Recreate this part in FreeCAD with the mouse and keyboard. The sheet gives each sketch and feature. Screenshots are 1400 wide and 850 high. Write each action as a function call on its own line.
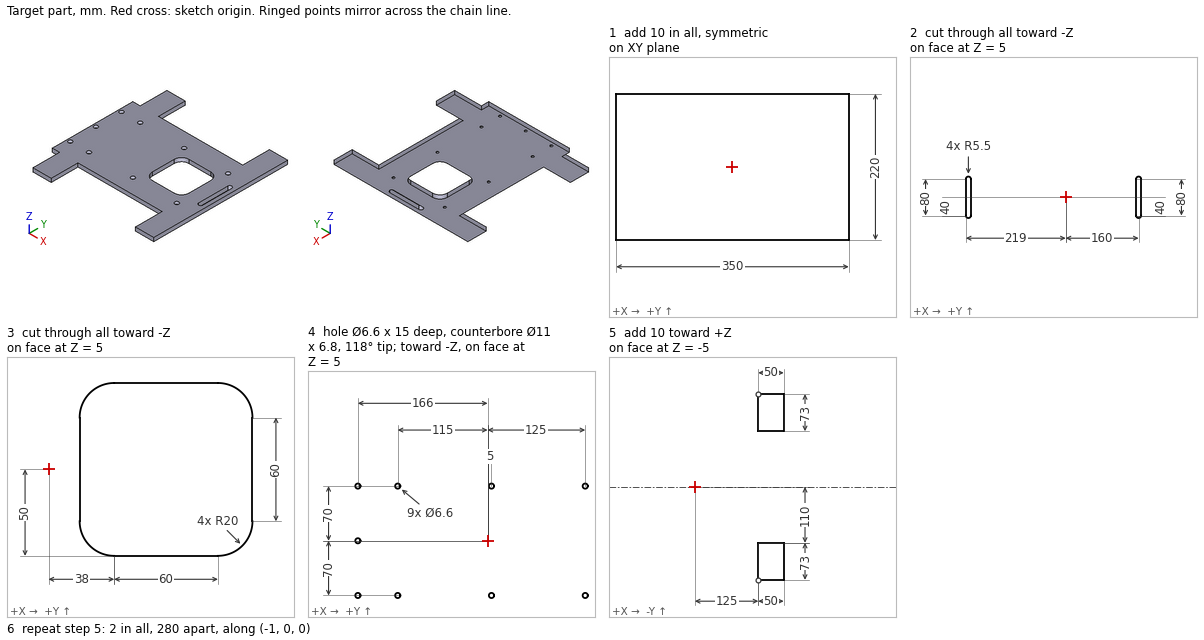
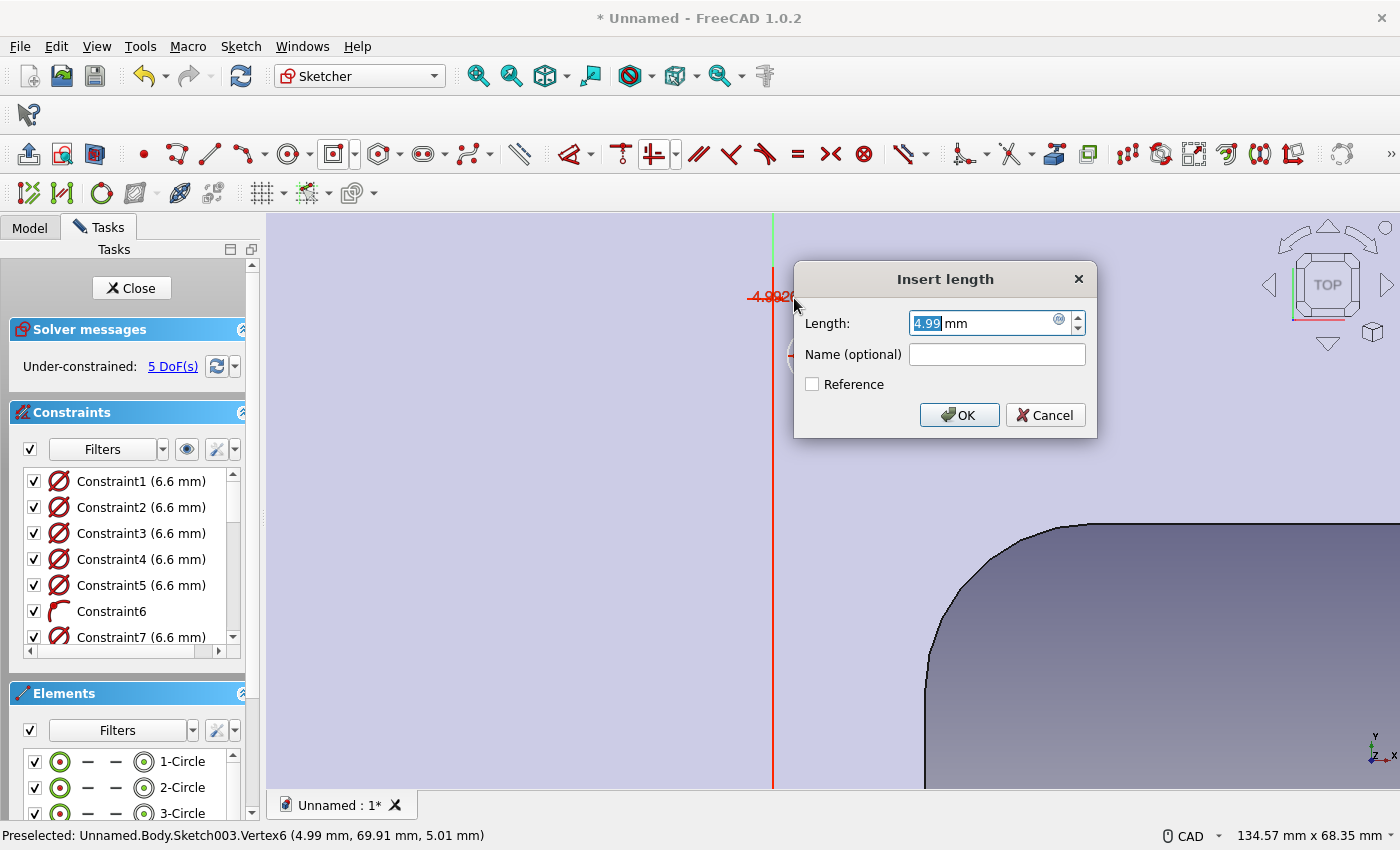
text(5)
key(Return)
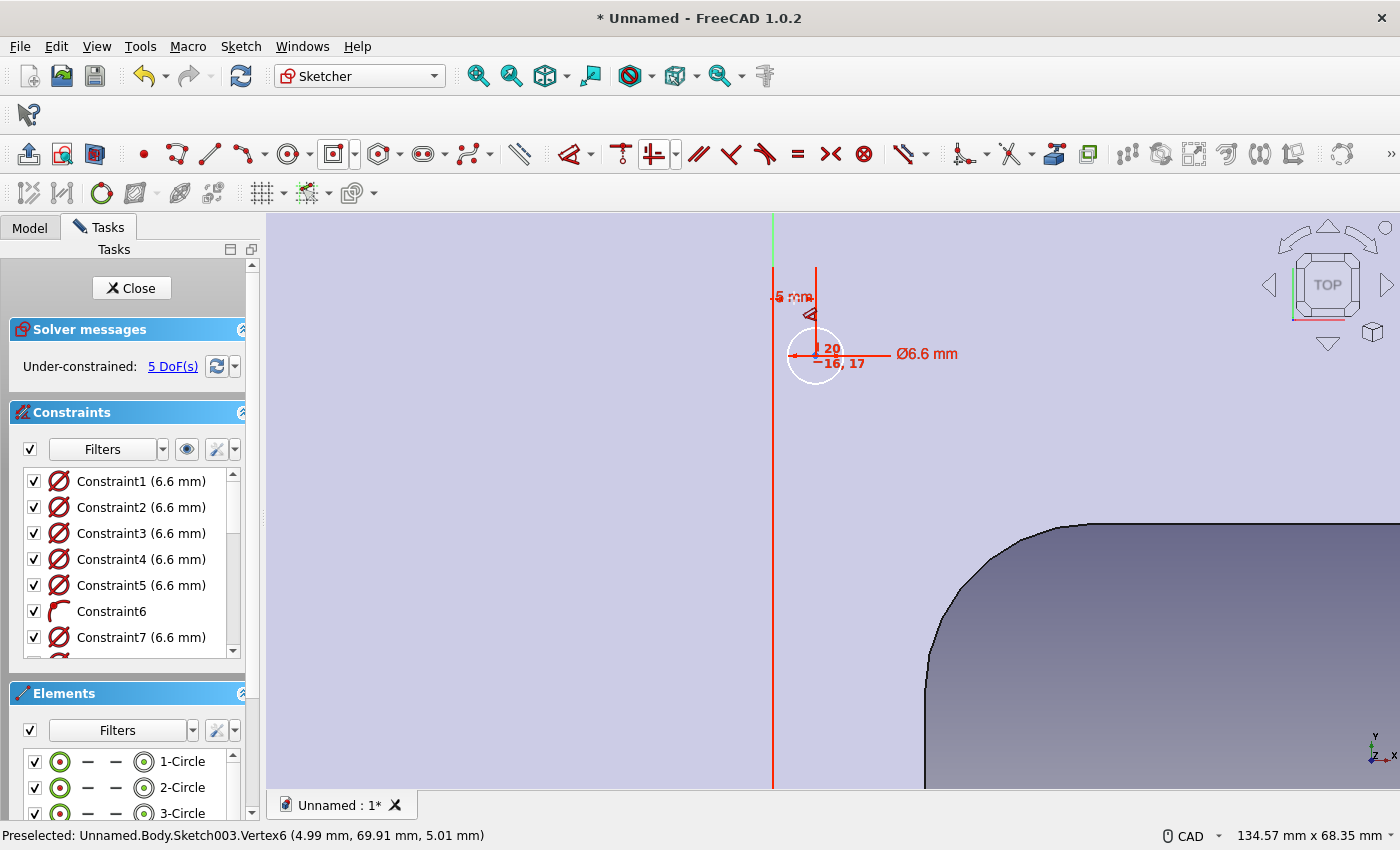
scroll(818, 356, down, 7)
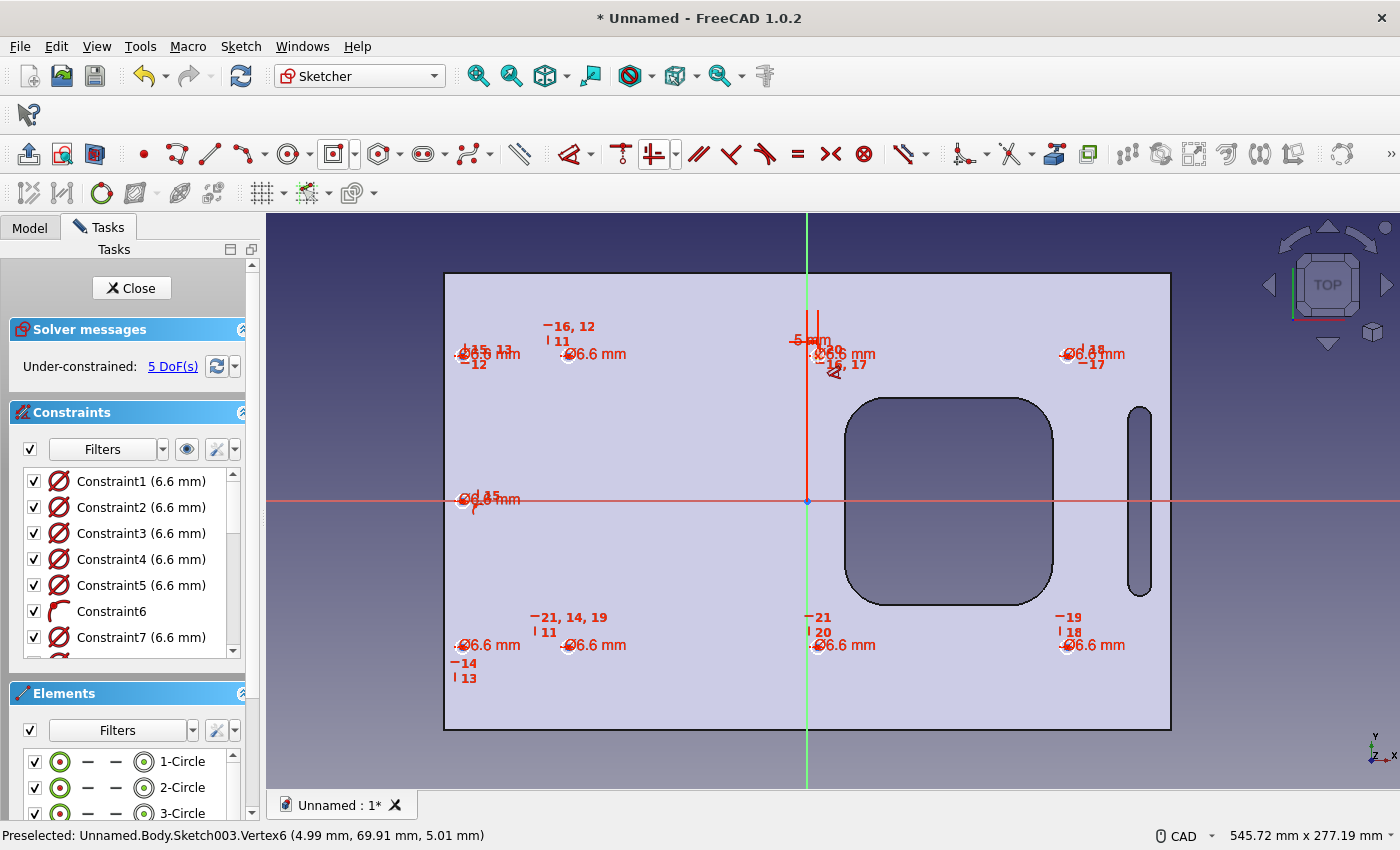
click(568, 356)
click(534, 429)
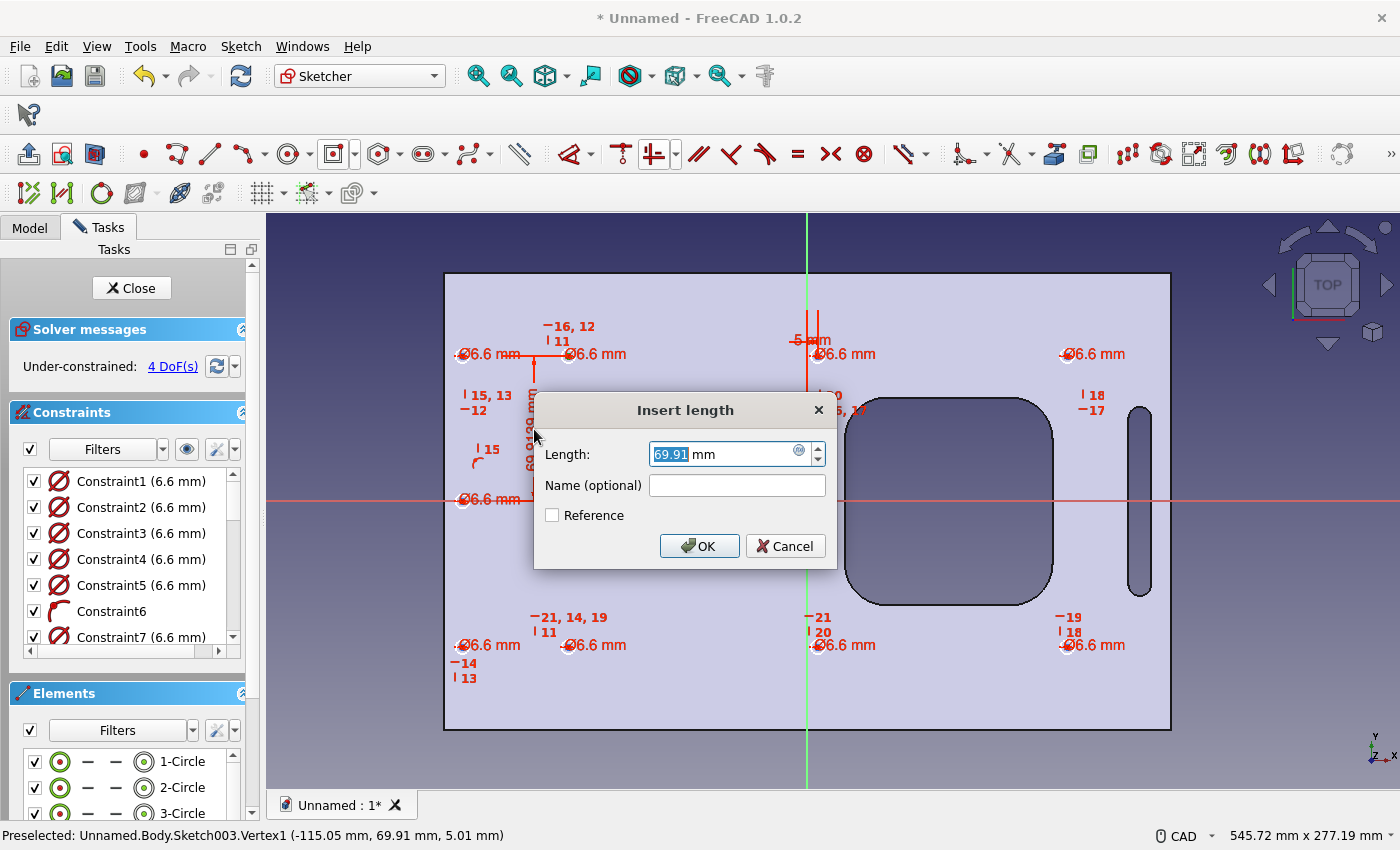
text(70)
key(Return)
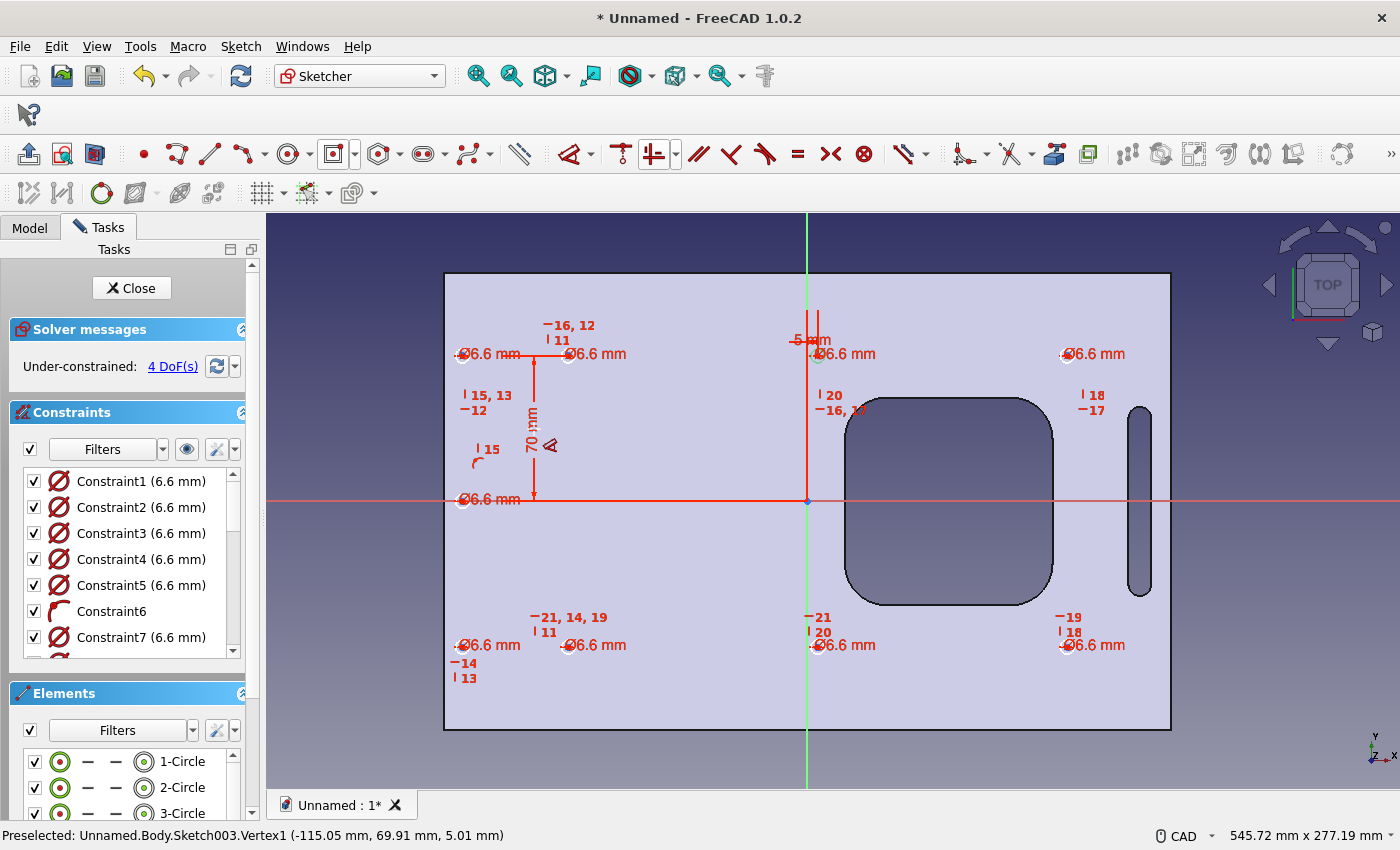
click(568, 647)
click(534, 574)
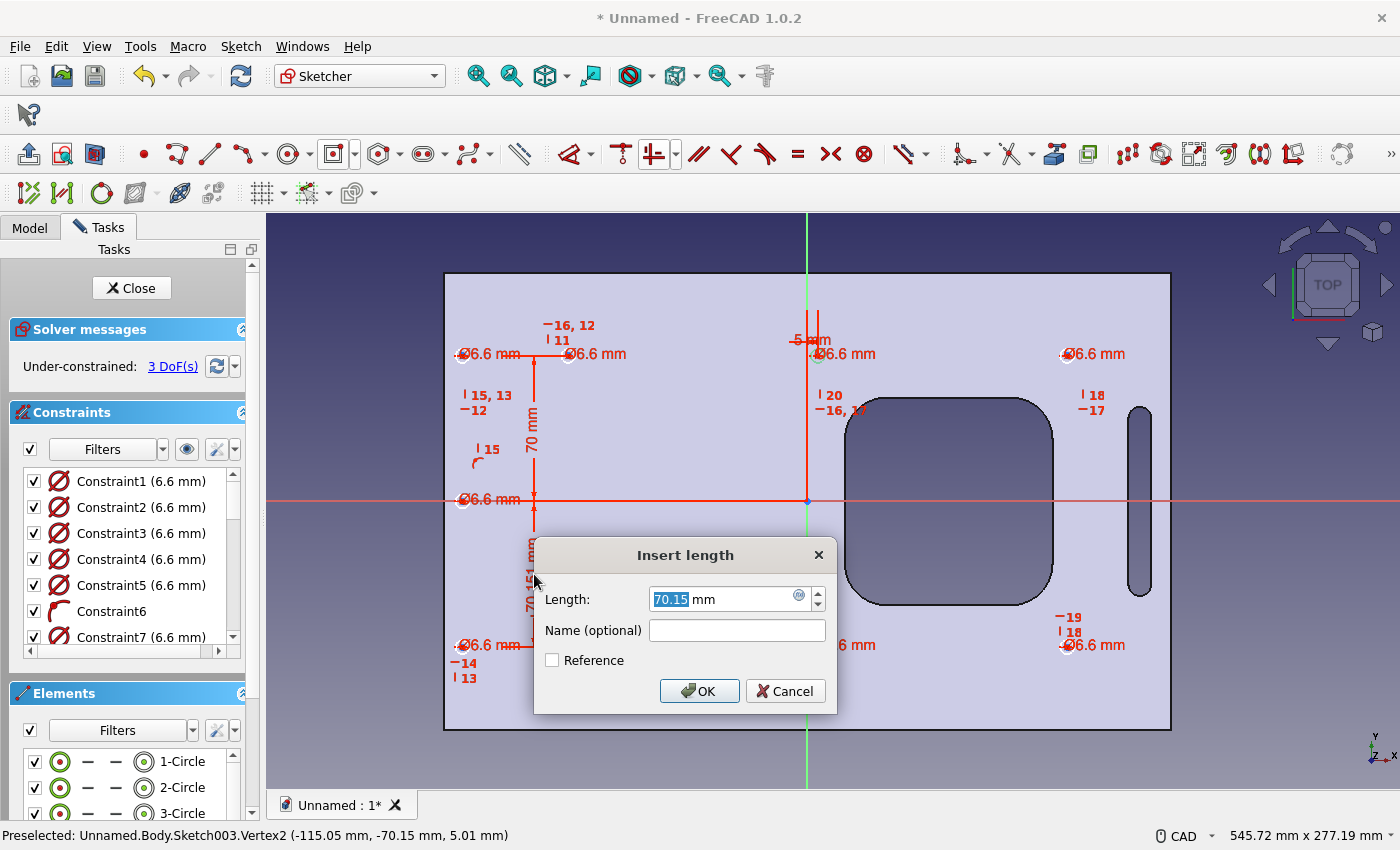
text(70)
key(Return)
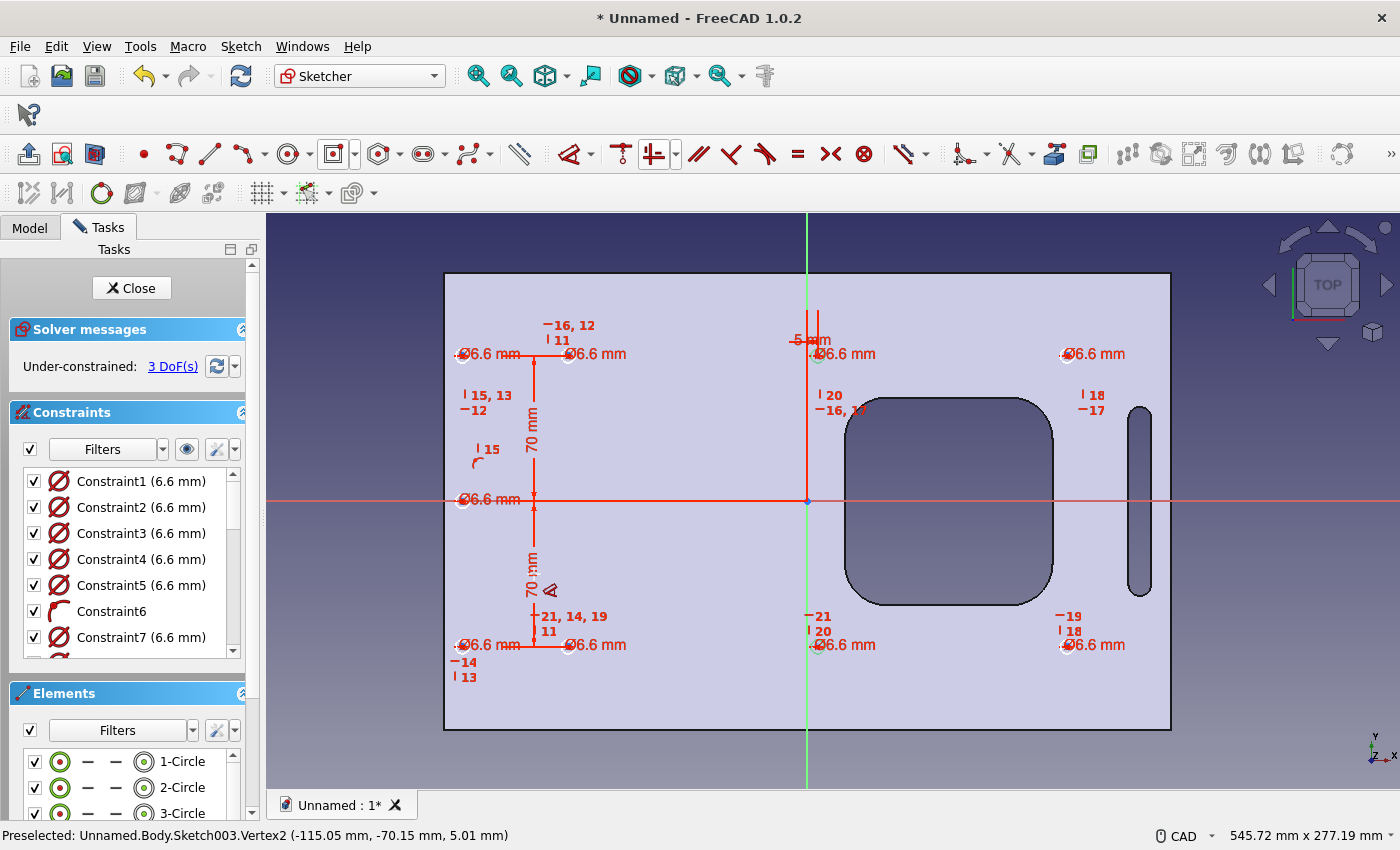
click(568, 356)
click(688, 322)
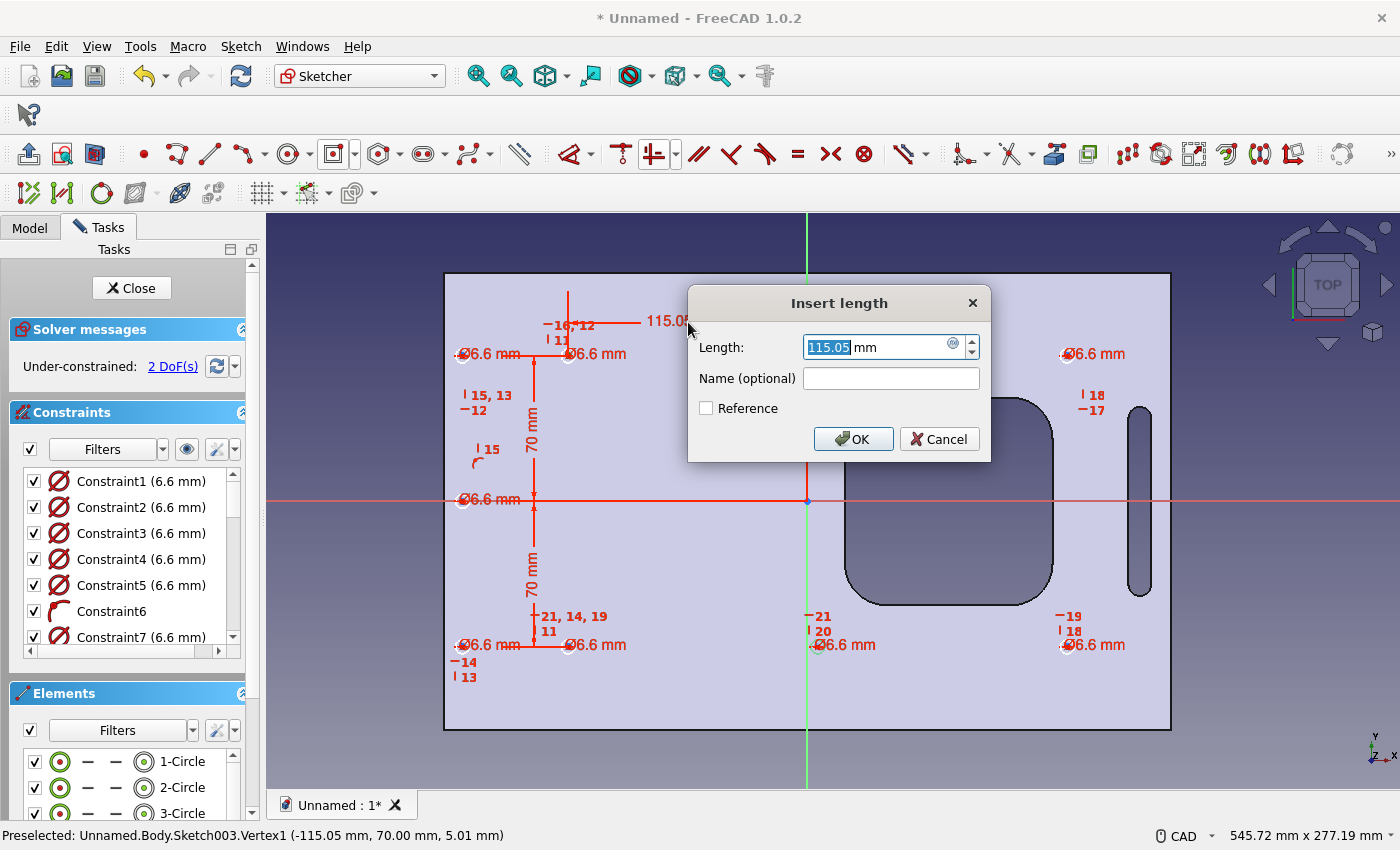
text(115)
key(Return)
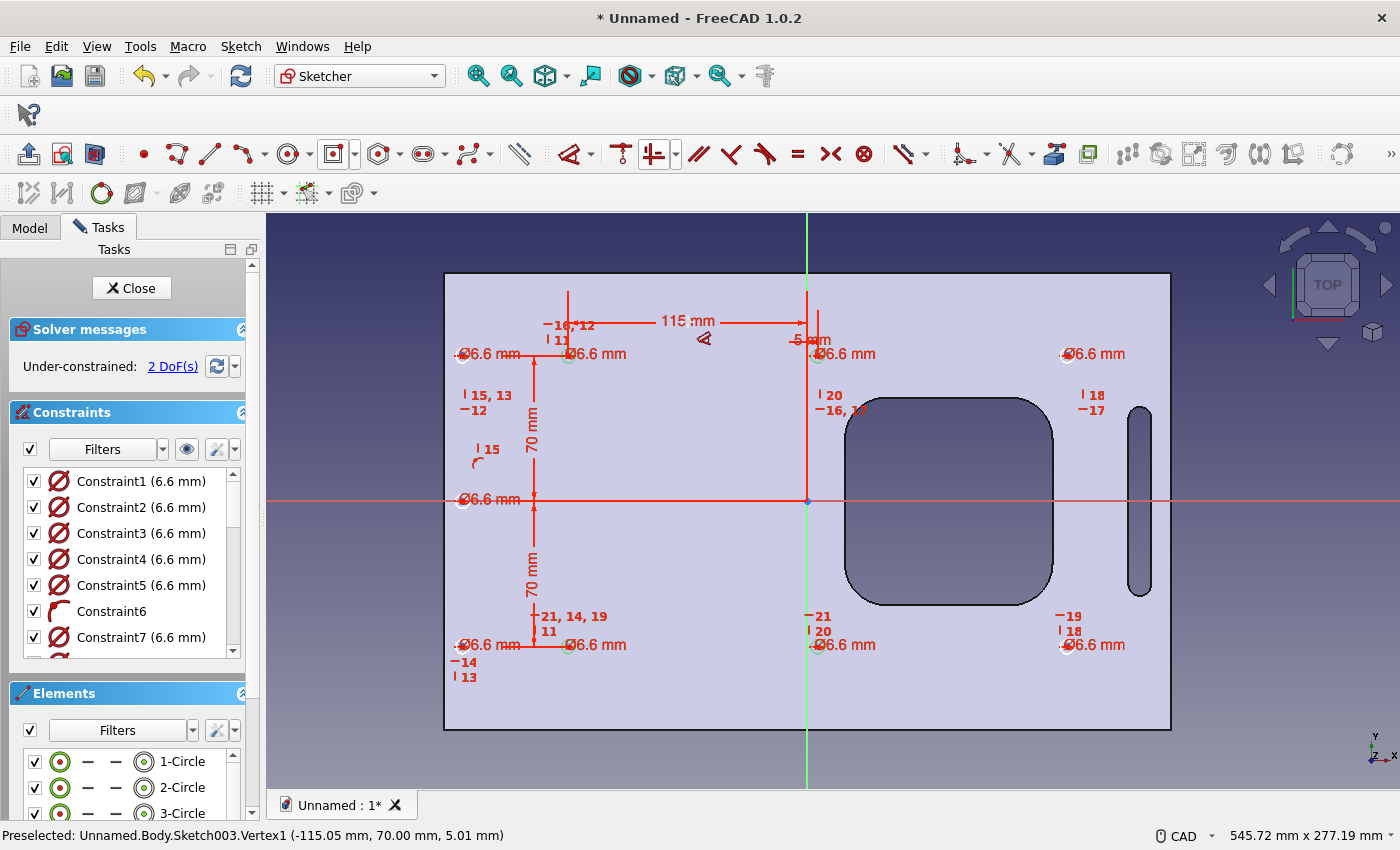
click(462, 356)
click(556, 322)